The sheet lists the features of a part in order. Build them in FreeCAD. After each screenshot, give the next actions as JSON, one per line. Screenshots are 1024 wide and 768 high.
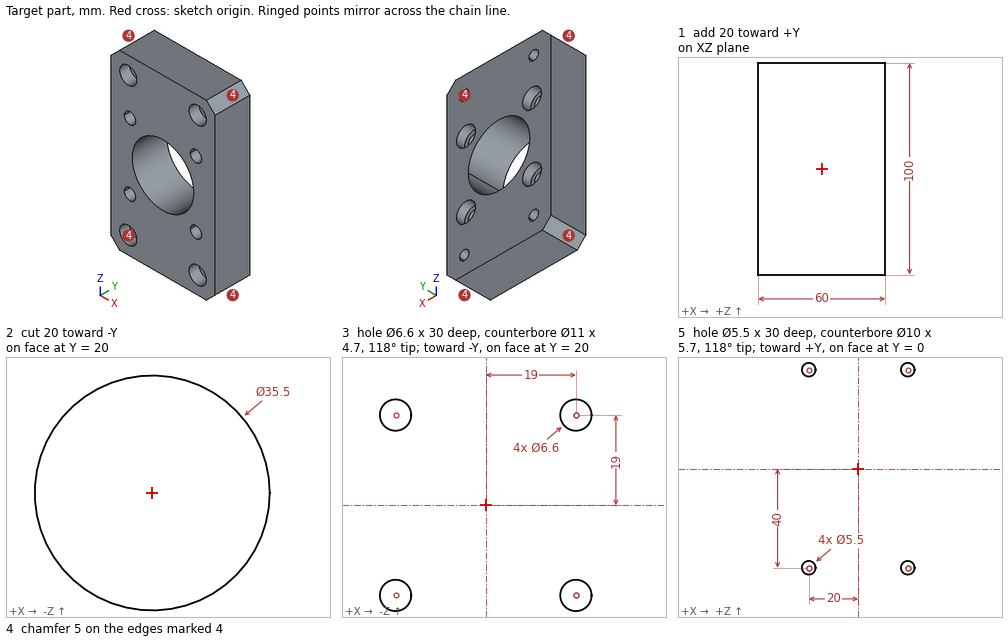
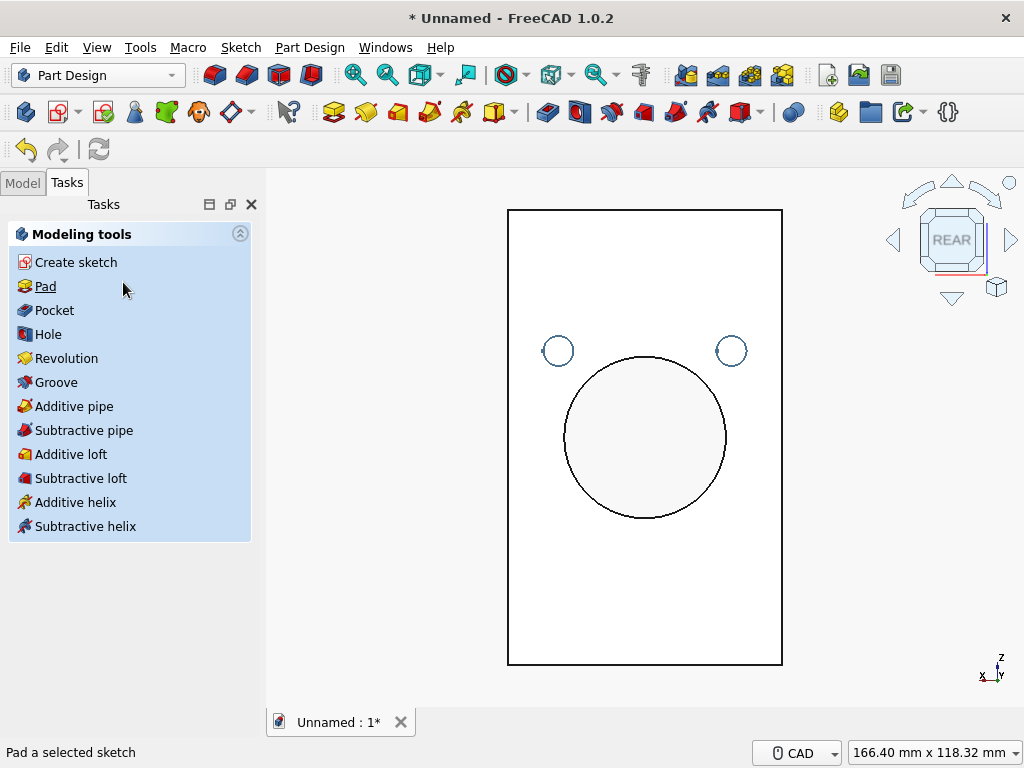
{"action": "left_click", "coordinate": [580, 112]}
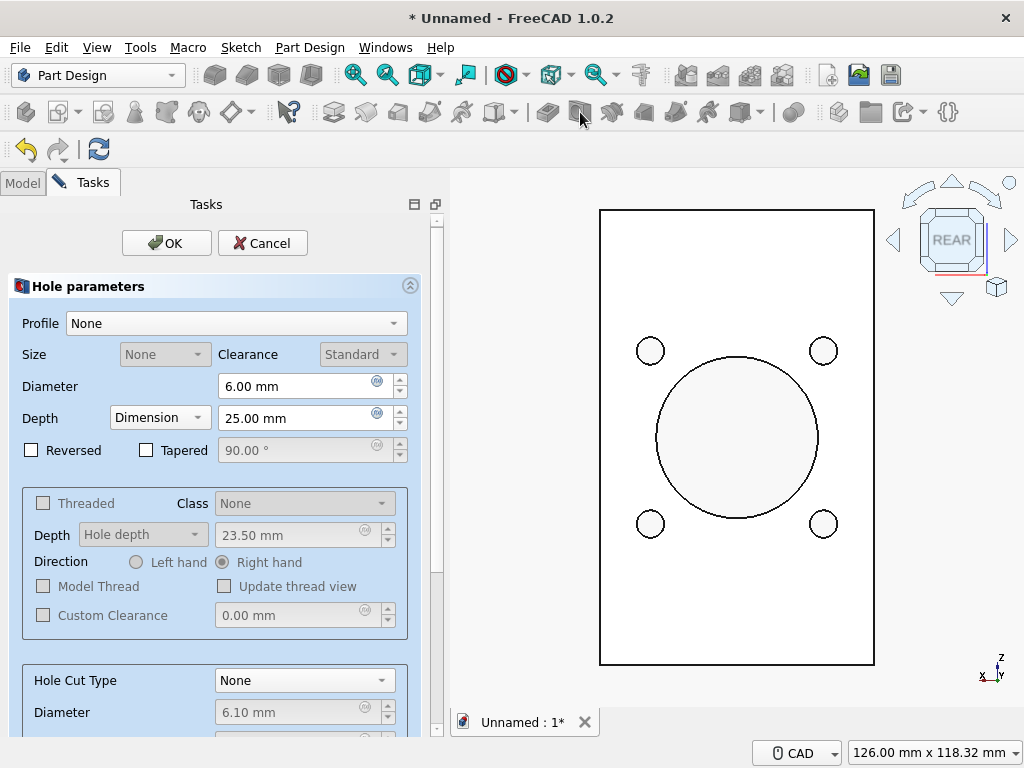
{"action": "triple_click", "coordinate": [305, 386]}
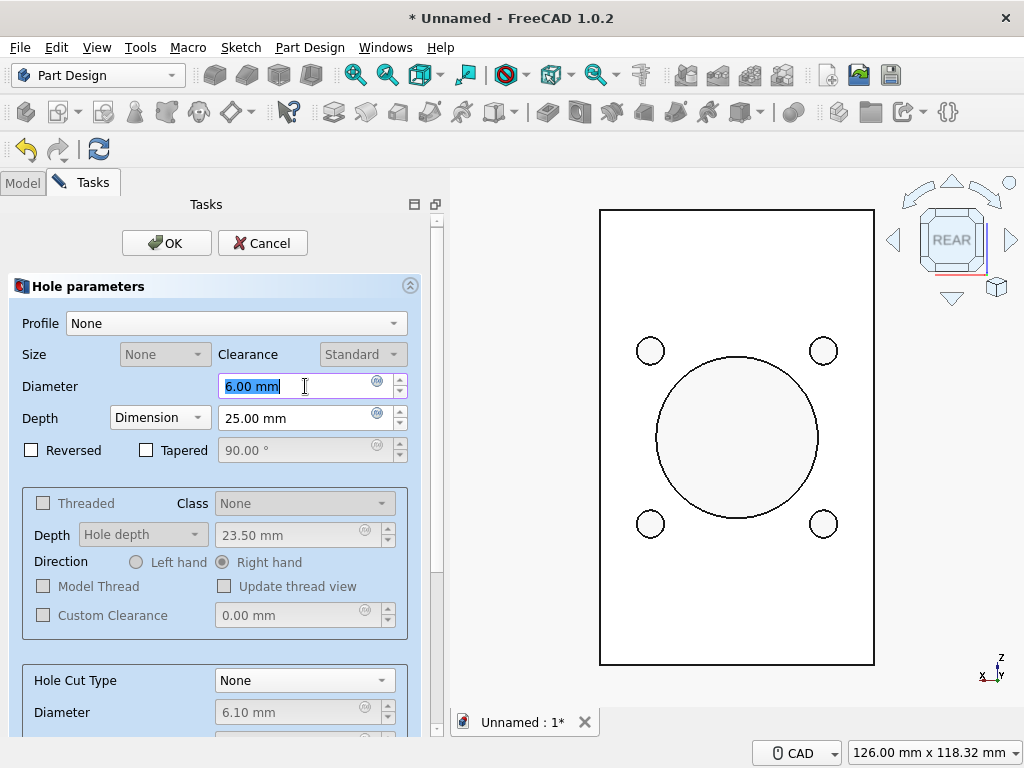
{"action": "type", "text": "6.6"}
{"action": "key", "text": "Tab"}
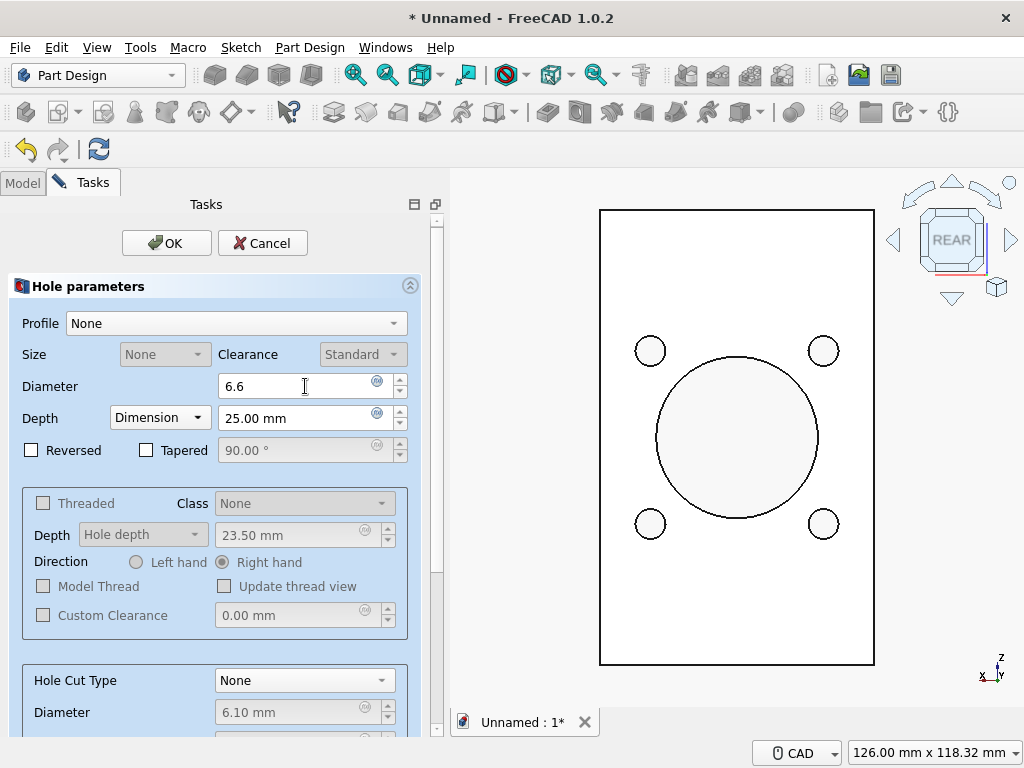
{"action": "triple_click", "coordinate": [305, 418]}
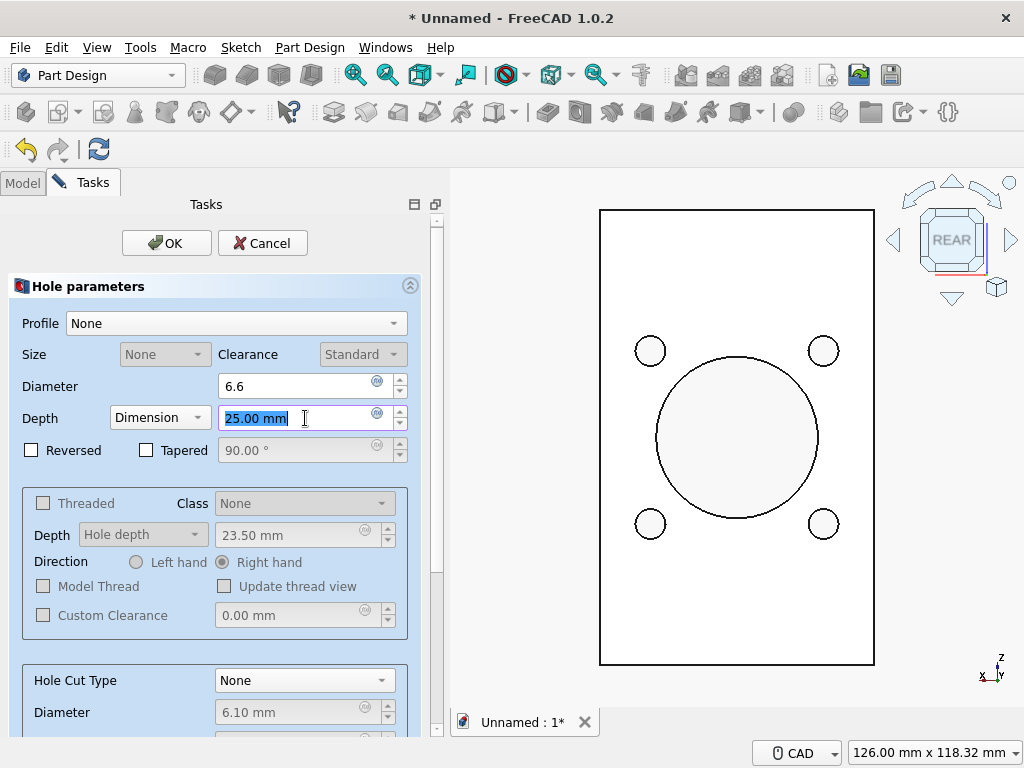
{"action": "type", "text": "30"}
{"action": "key", "text": "Tab"}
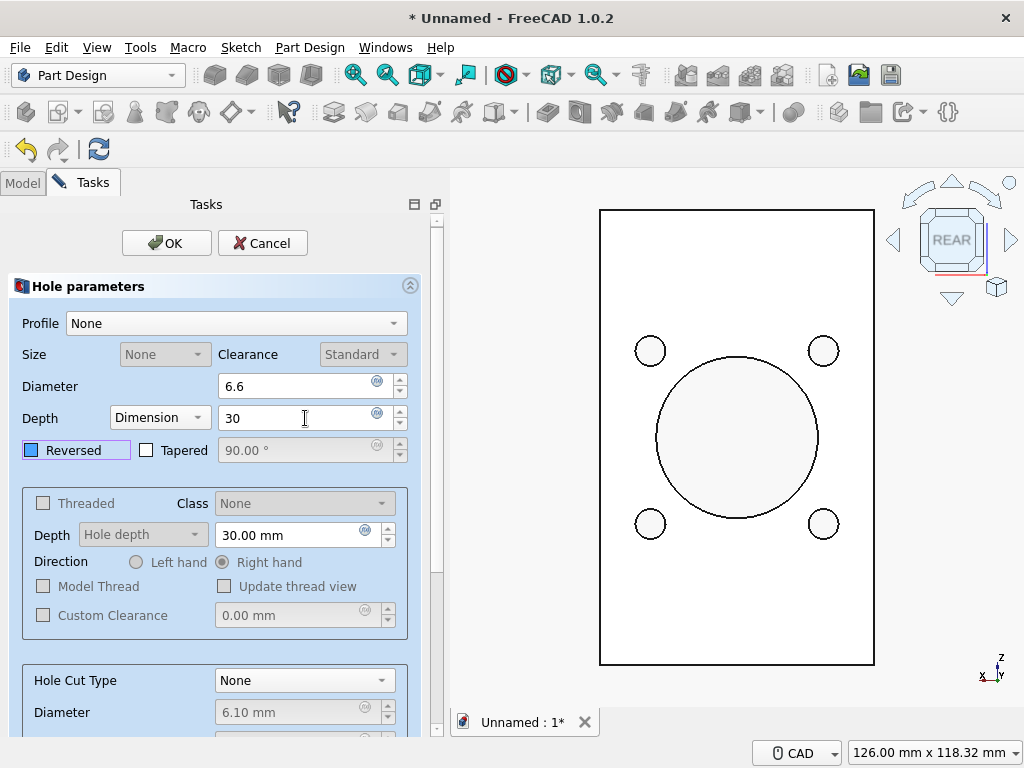
{"action": "left_click", "coordinate": [306, 680]}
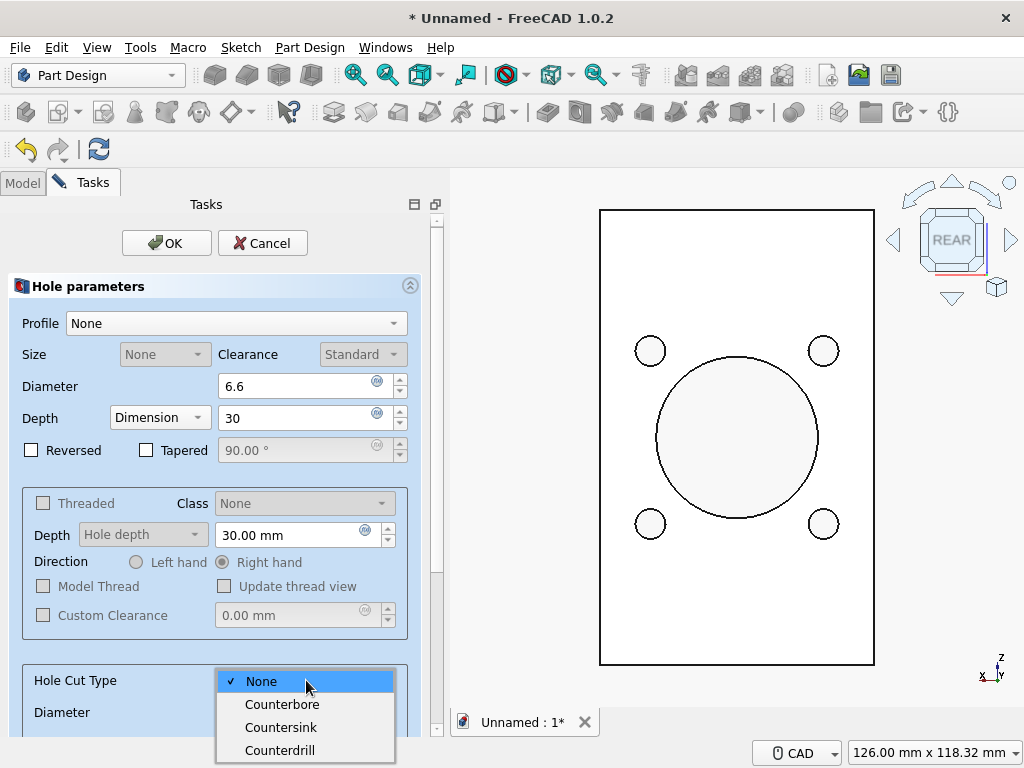
{"action": "left_click", "coordinate": [304, 704]}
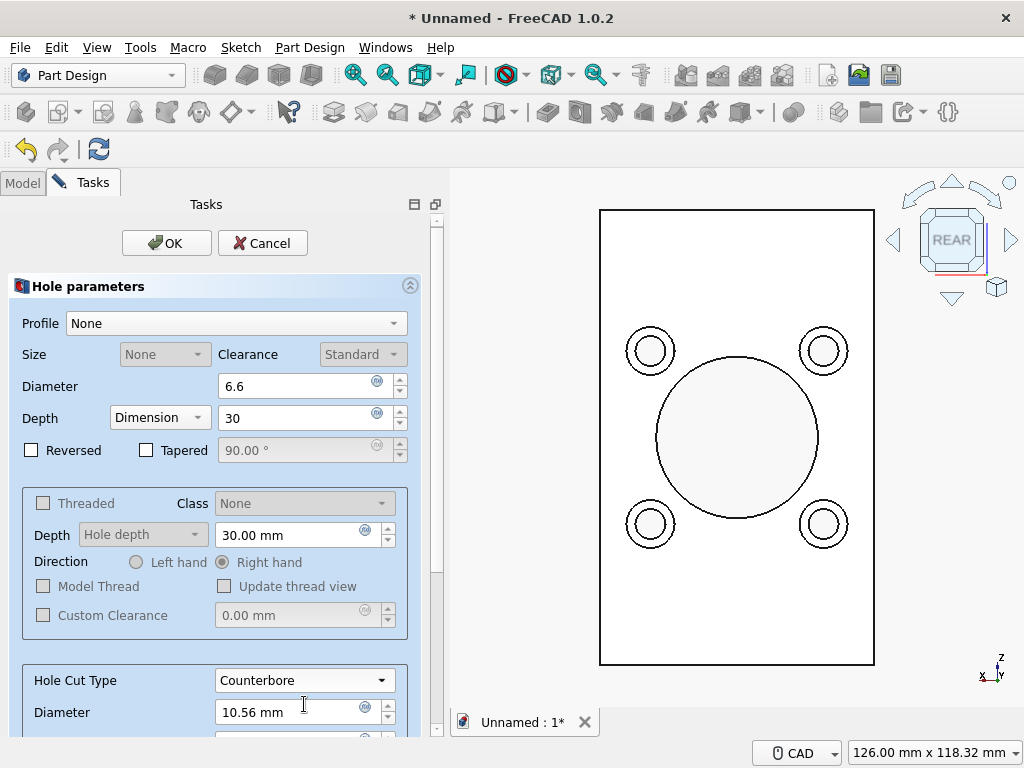
{"action": "triple_click", "coordinate": [298, 712]}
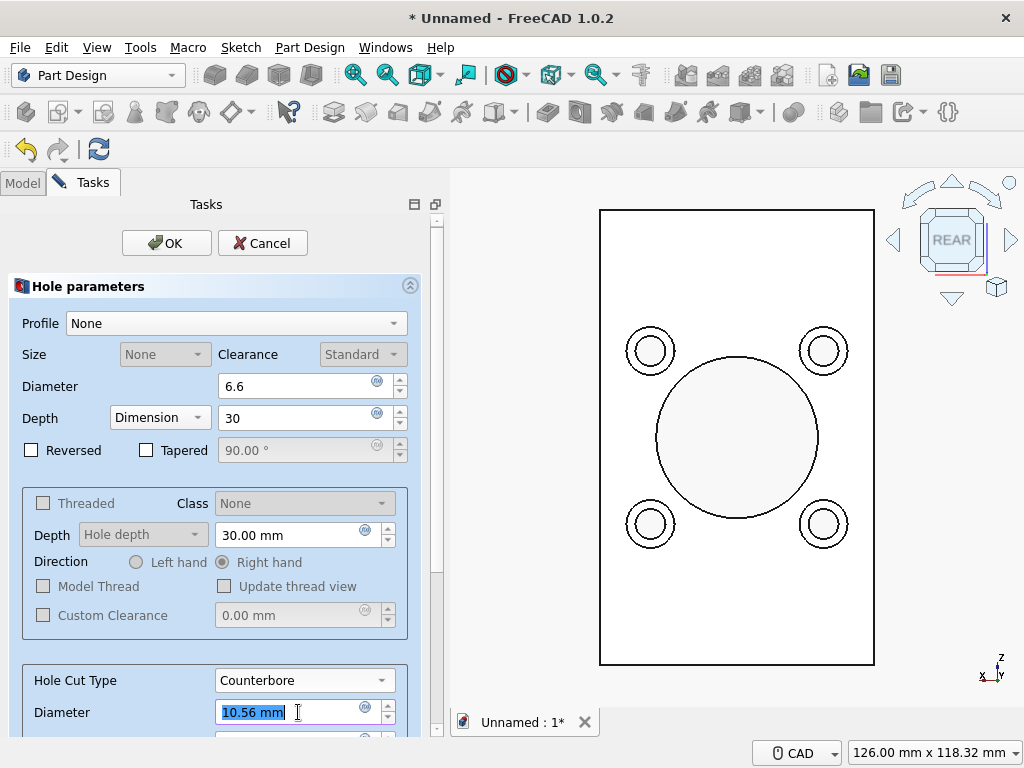
{"action": "type", "text": "11"}
{"action": "key", "text": "Tab"}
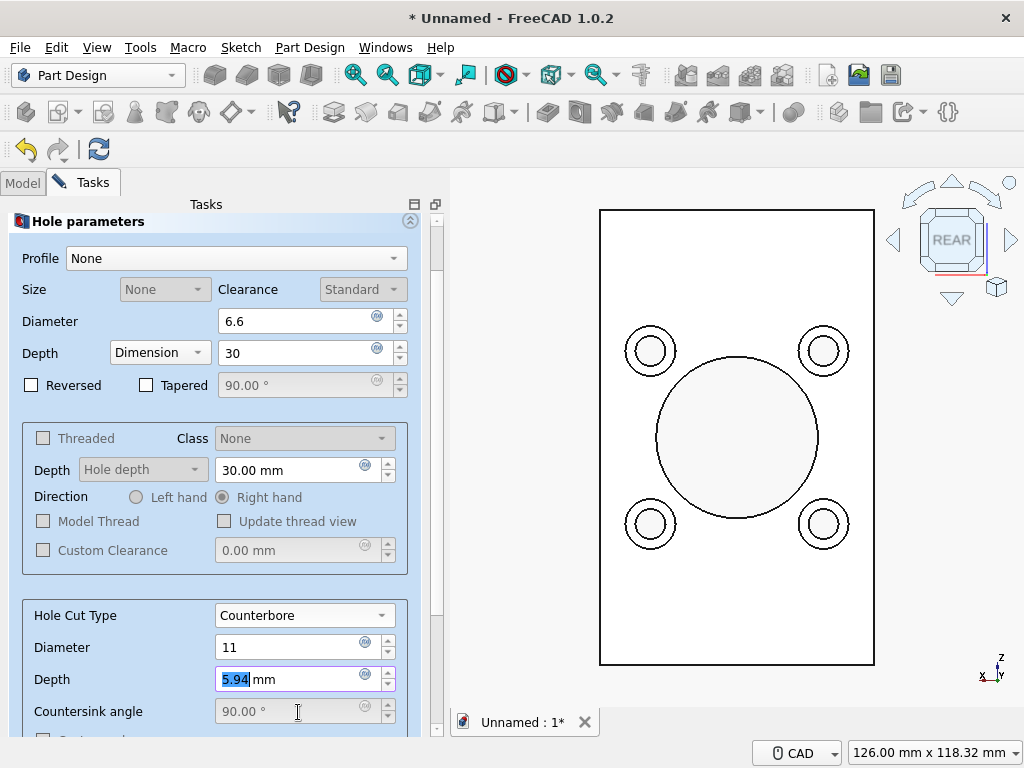
{"action": "type", "text": "4.7"}
{"action": "key", "text": "Tab"}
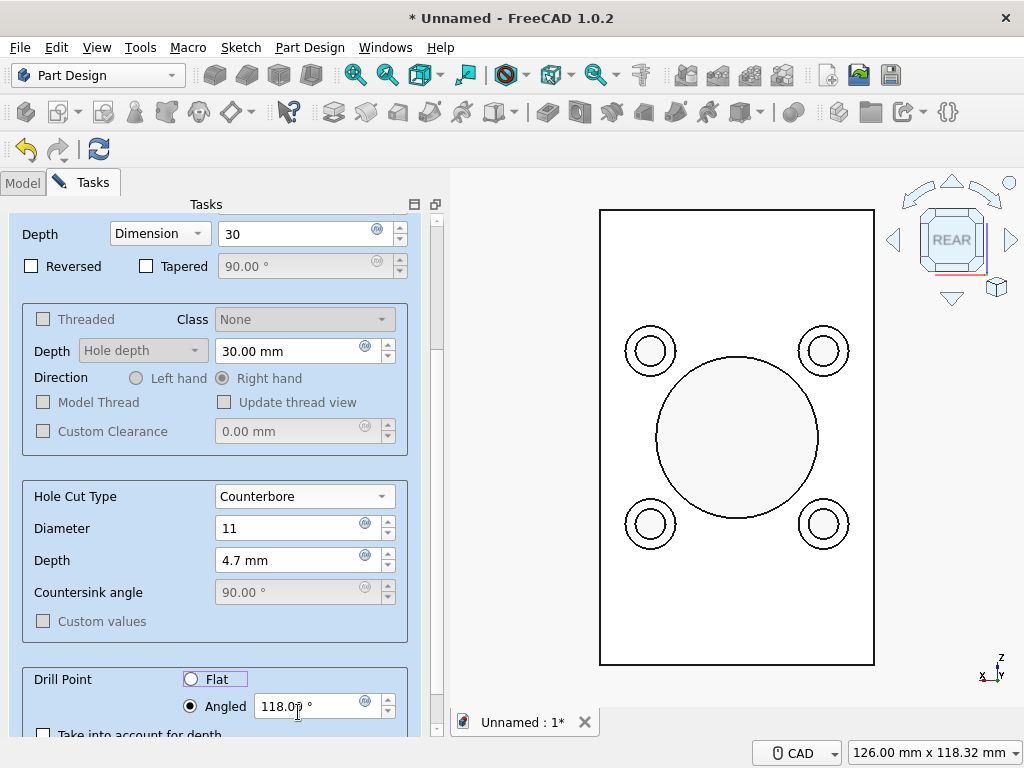
{"action": "scroll", "coordinate": [437, 475], "scroll_direction": "up", "scroll_amount": 4}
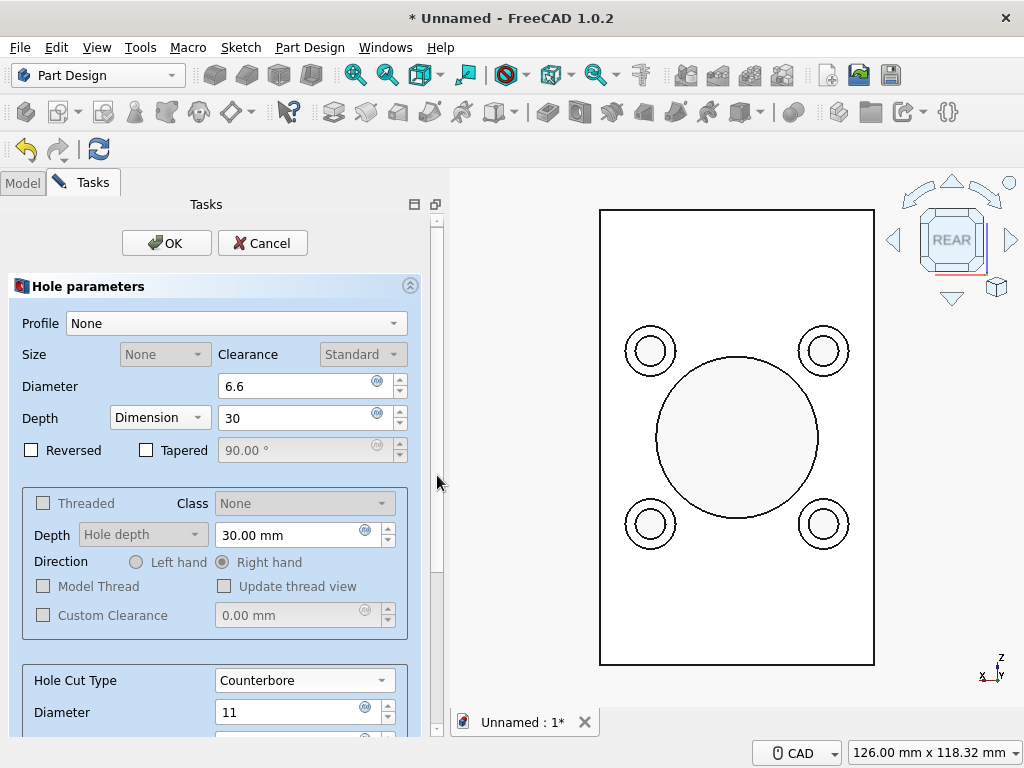
{"action": "left_click", "coordinate": [167, 243]}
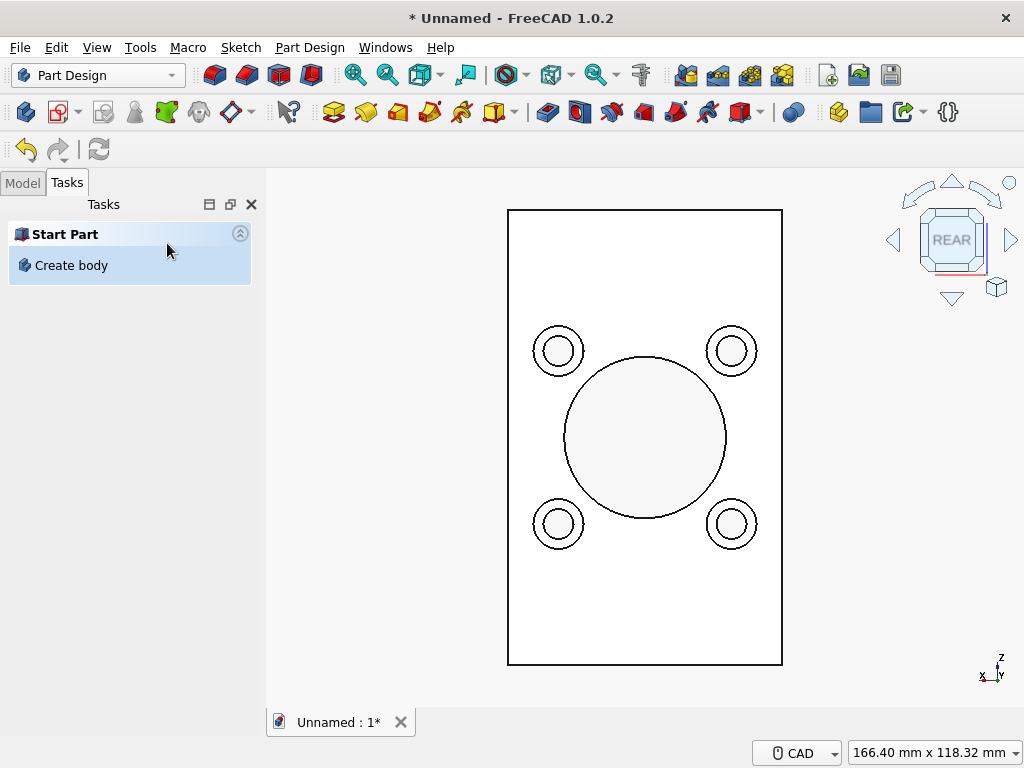
{"action": "key", "text": "0"}